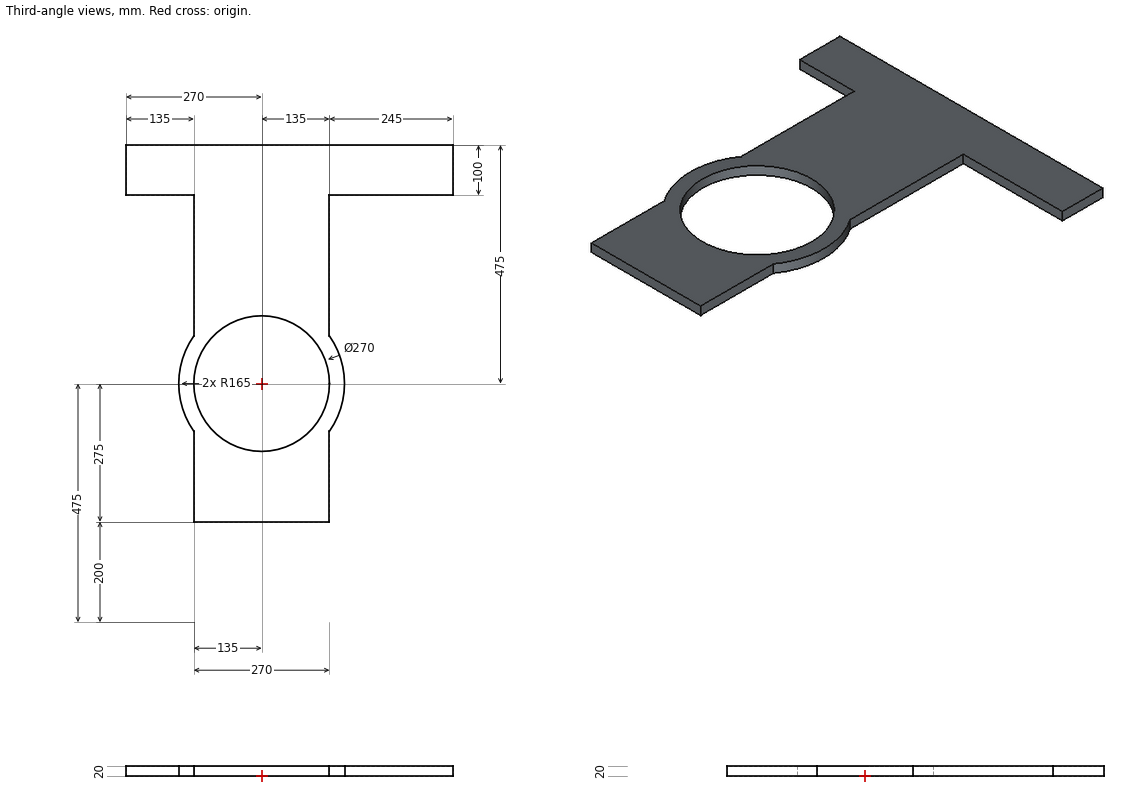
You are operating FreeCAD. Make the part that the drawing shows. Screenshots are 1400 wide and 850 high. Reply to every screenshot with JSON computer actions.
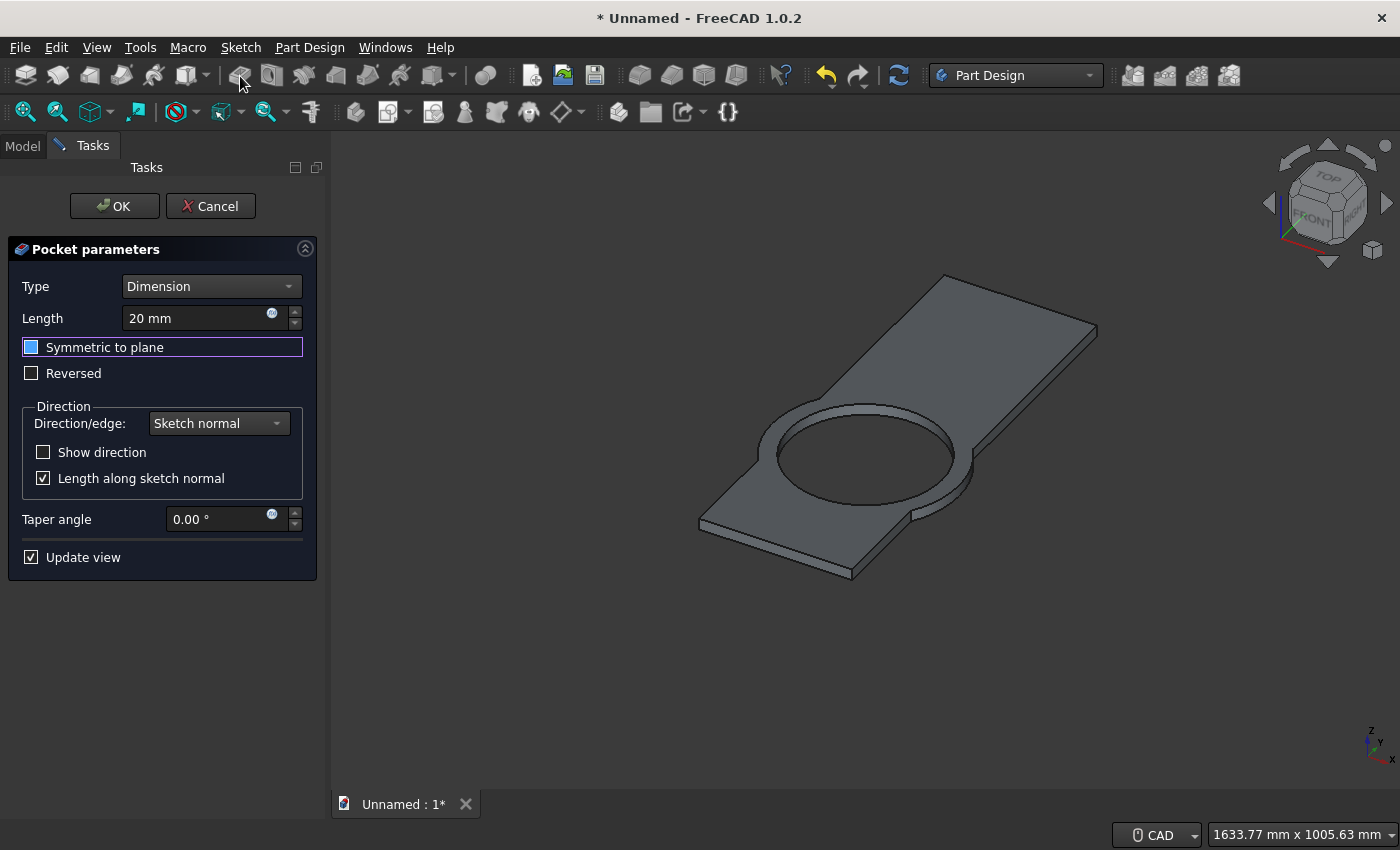
{"action": "left_click", "coordinate": [115, 206]}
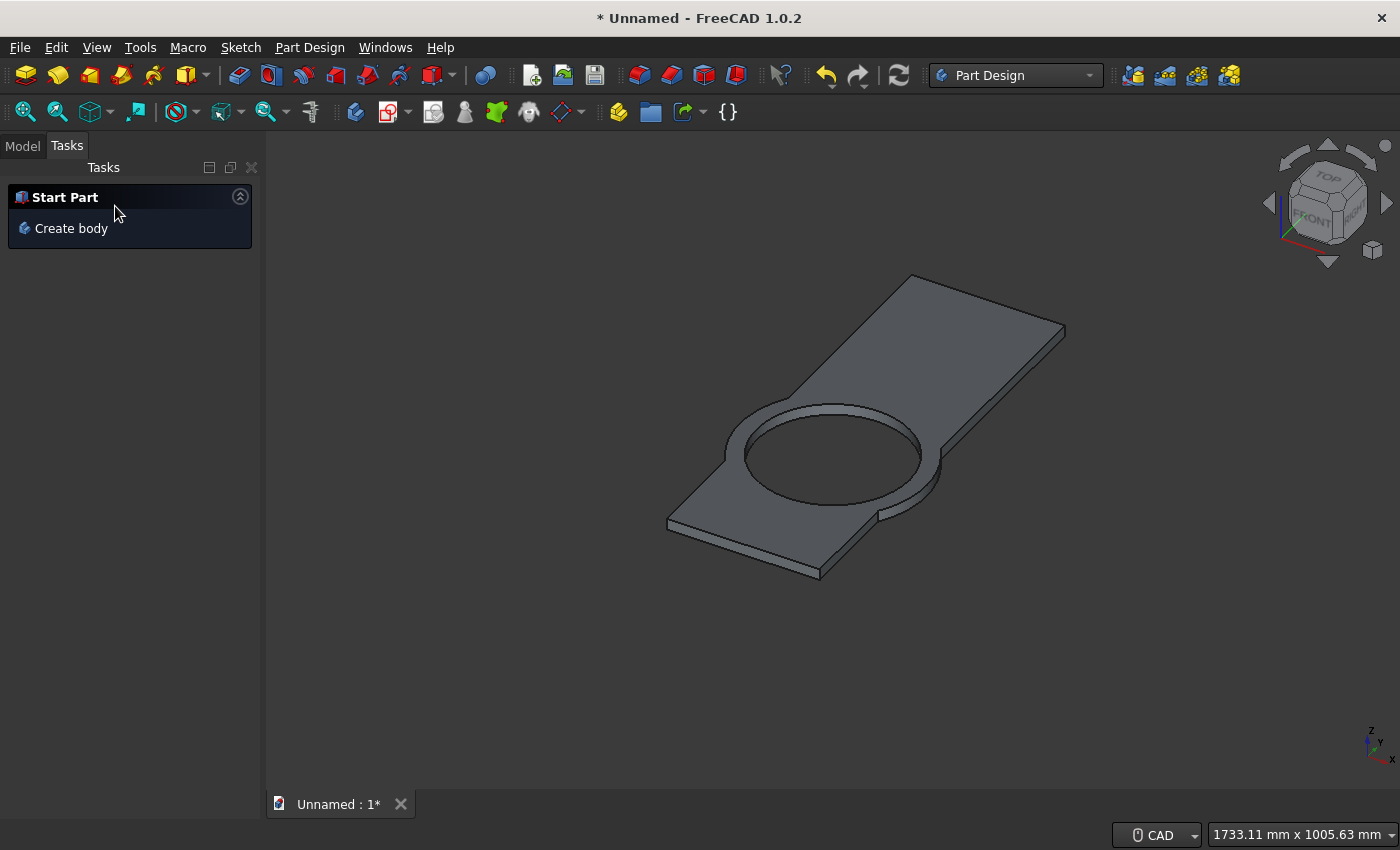
{"action": "left_click", "coordinate": [388, 112]}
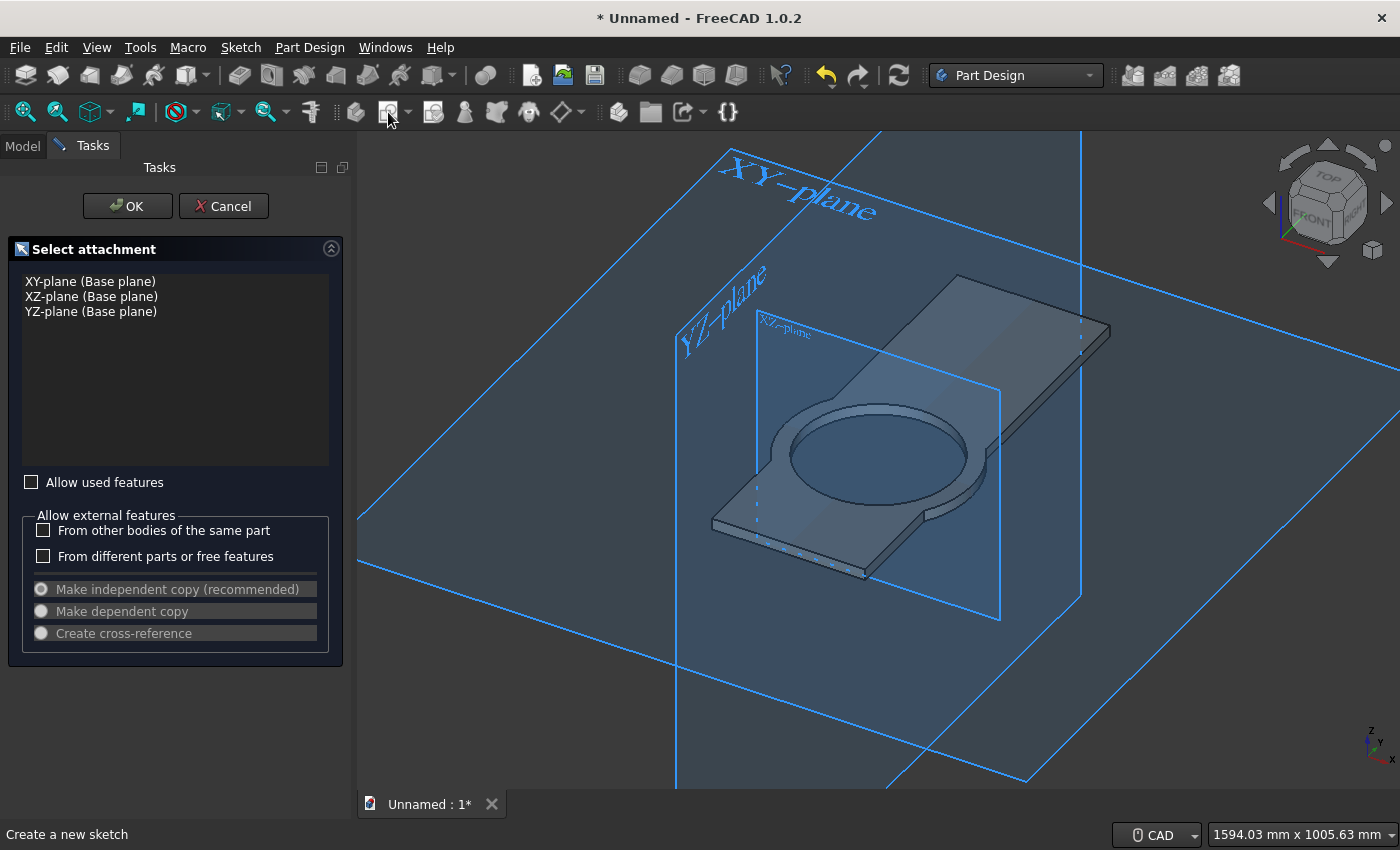
{"action": "left_click", "coordinate": [82, 282]}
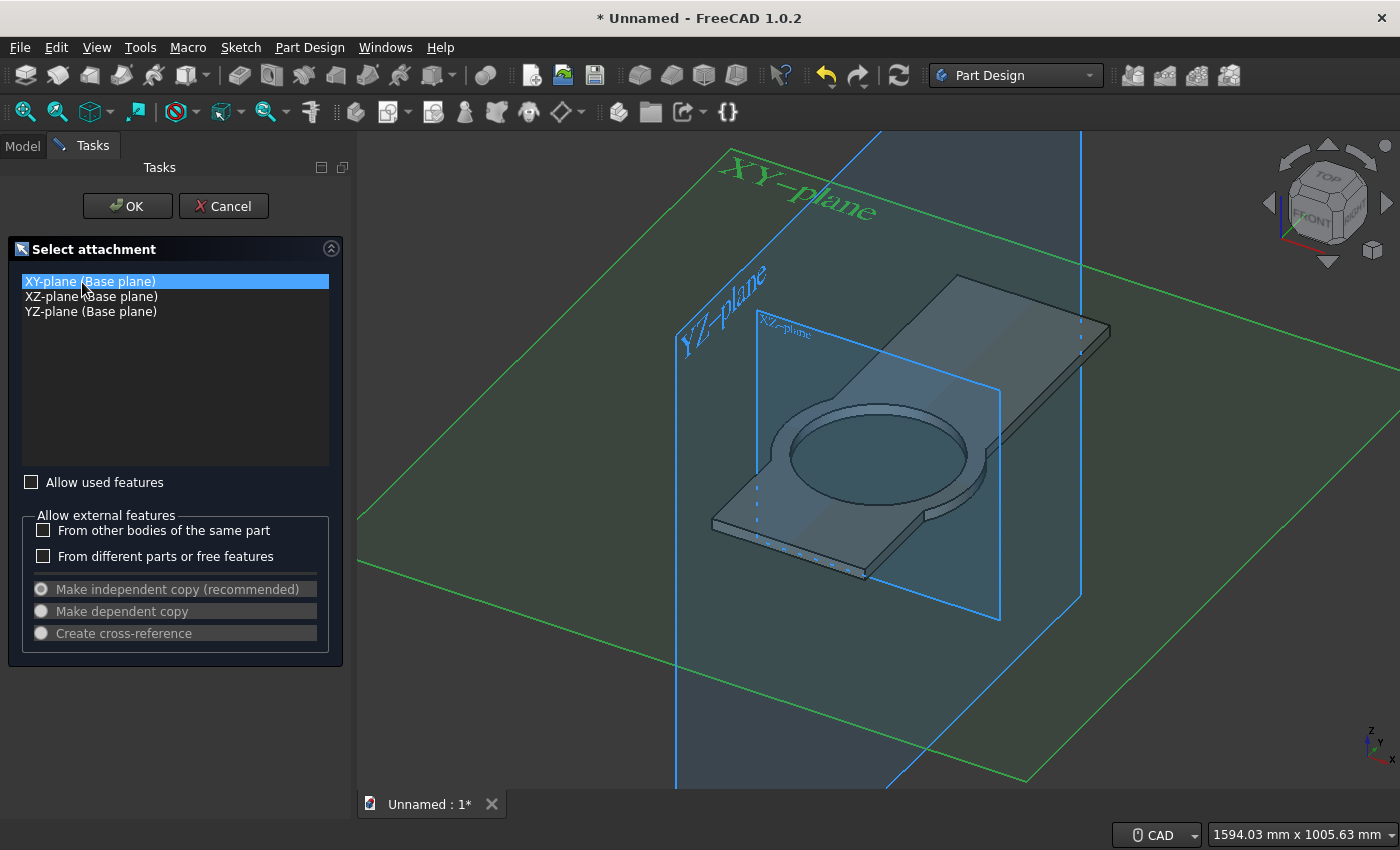
{"action": "left_click", "coordinate": [128, 206]}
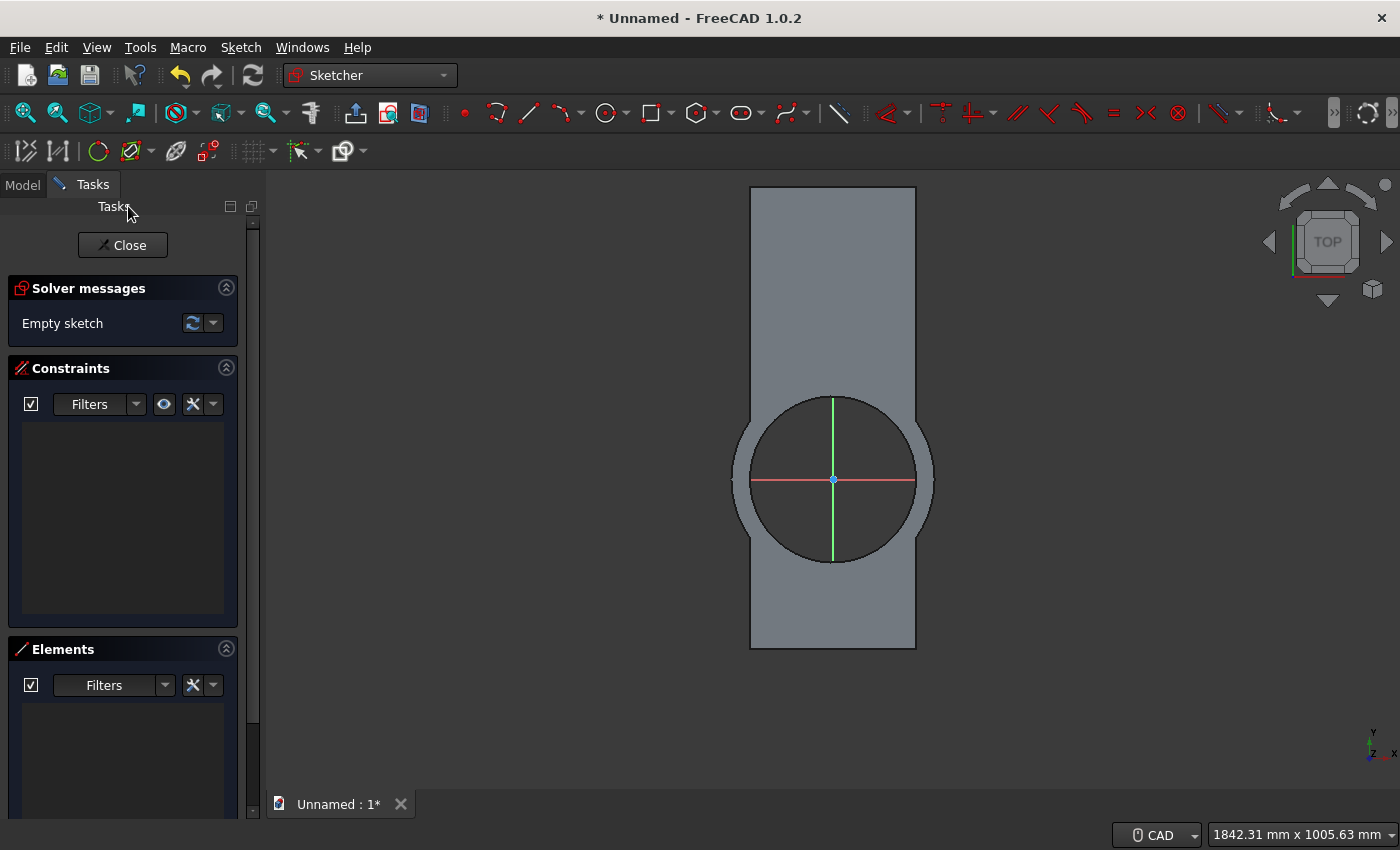
{"action": "left_click", "coordinate": [420, 114]}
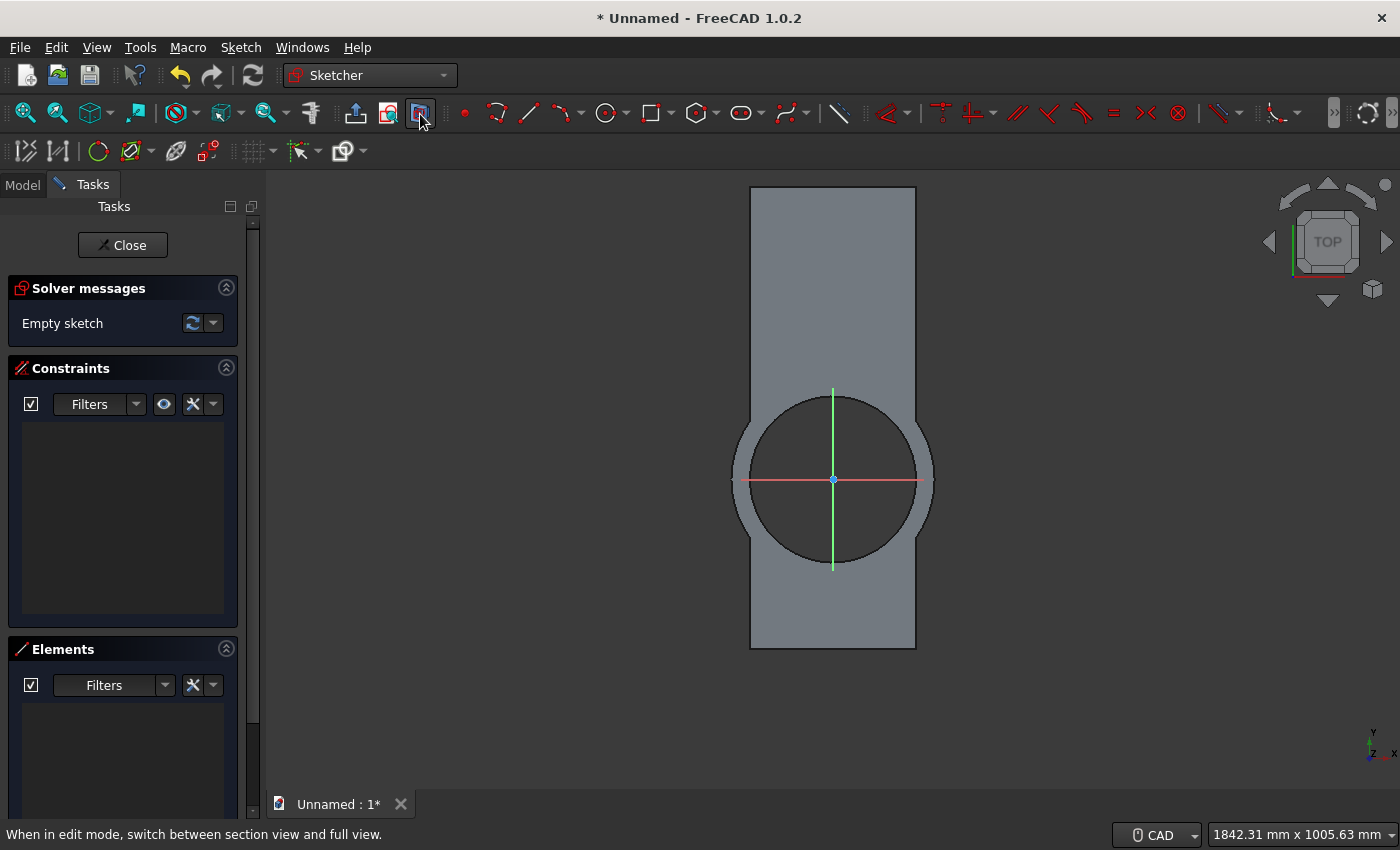
{"action": "scroll", "coordinate": [302, 761], "scroll_direction": "down", "scroll_amount": 1}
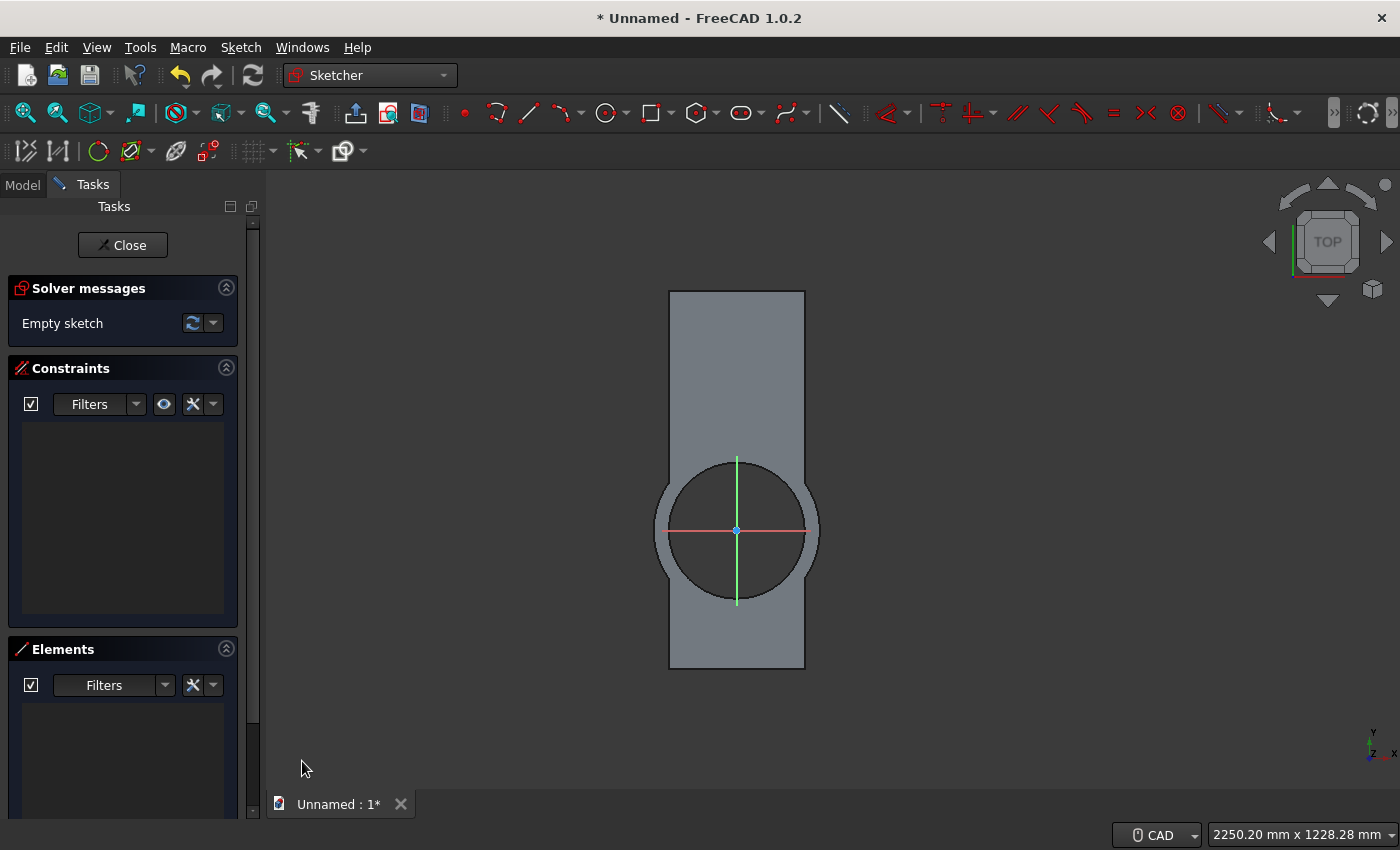
{"action": "scroll", "coordinate": [764, 328], "scroll_direction": "up", "scroll_amount": 3}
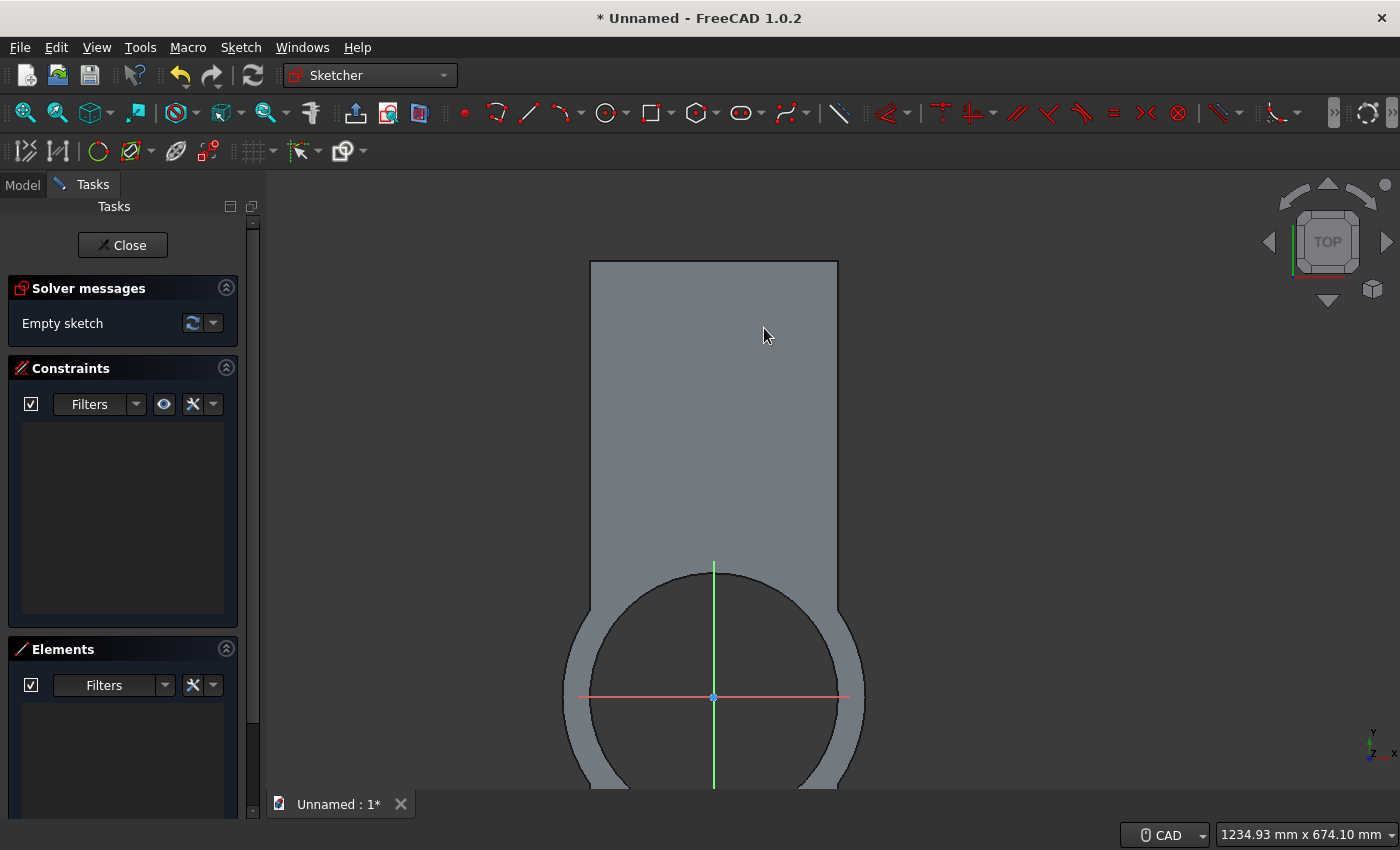
{"action": "left_click", "coordinate": [652, 114]}